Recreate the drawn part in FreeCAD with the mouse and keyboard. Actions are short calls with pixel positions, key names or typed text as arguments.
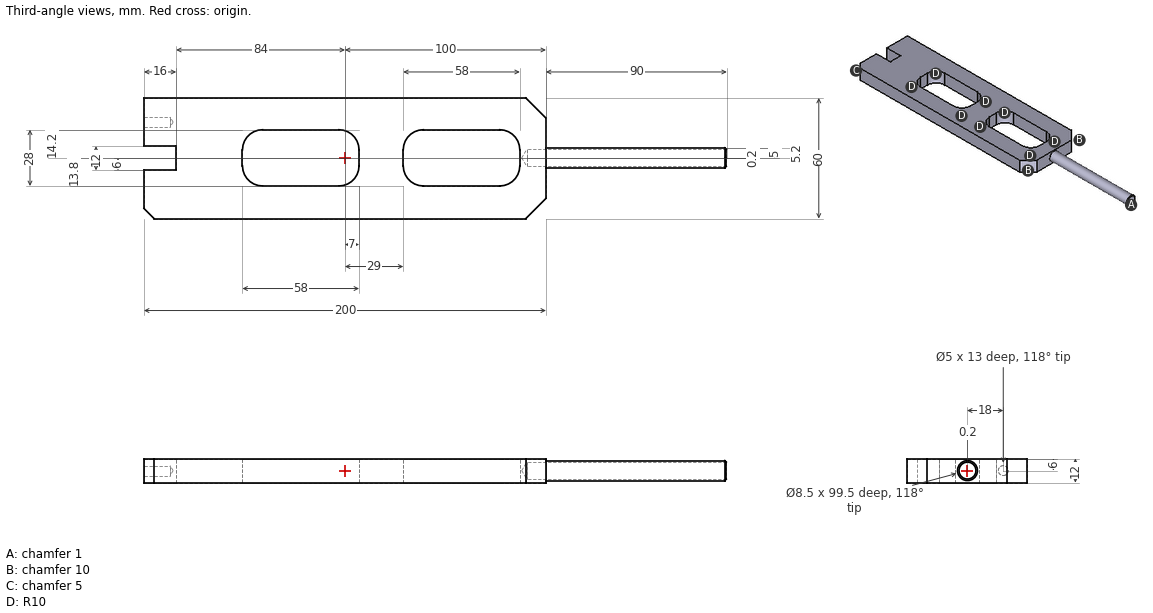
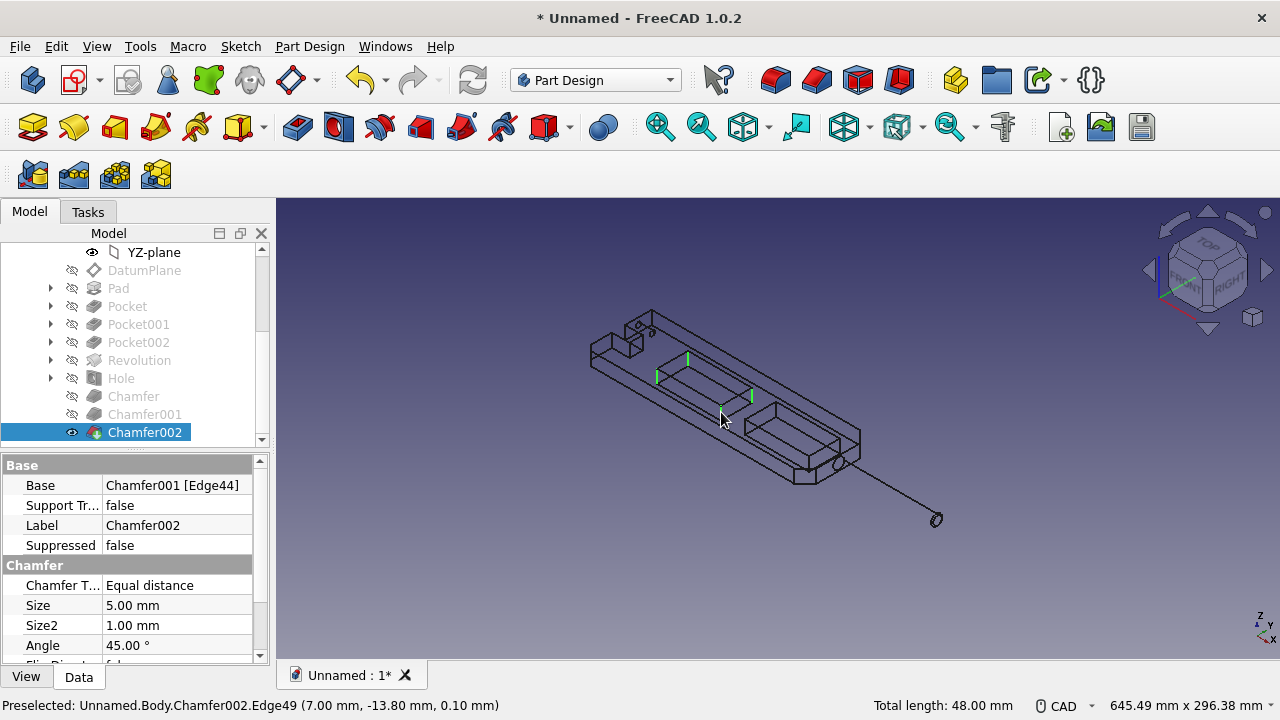
click(776, 410, ctrl)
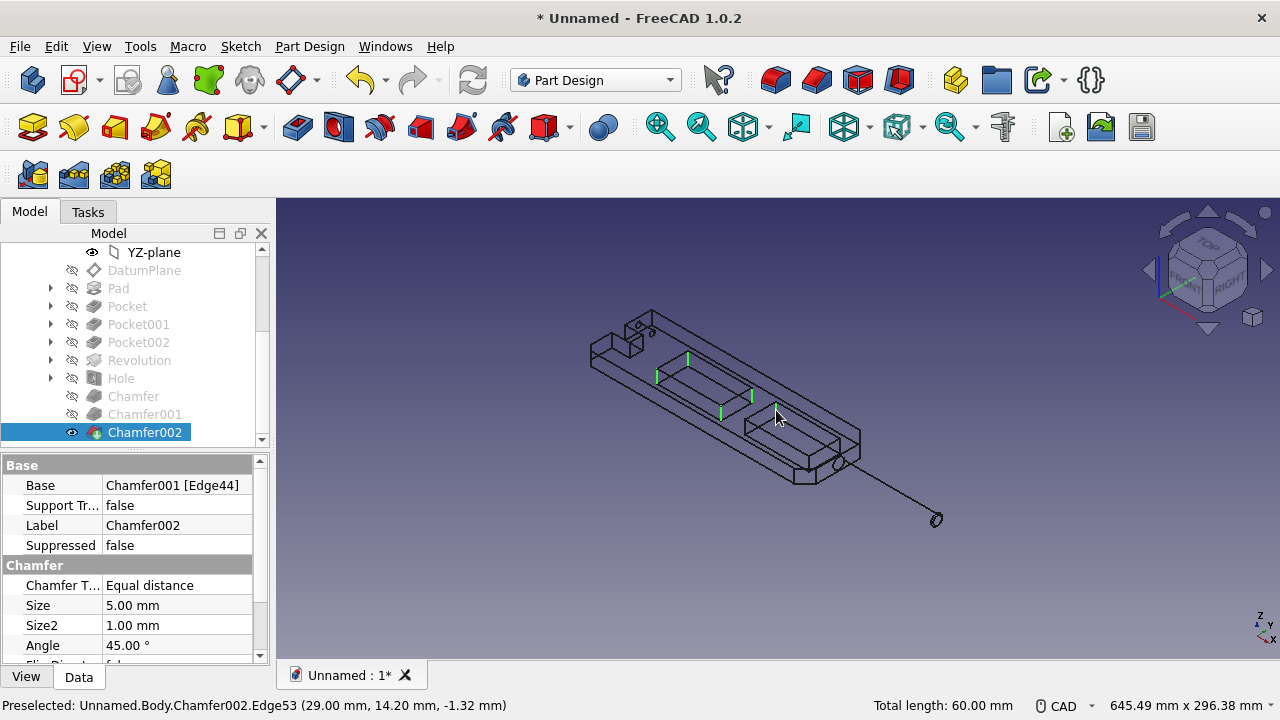
click(745, 426, ctrl)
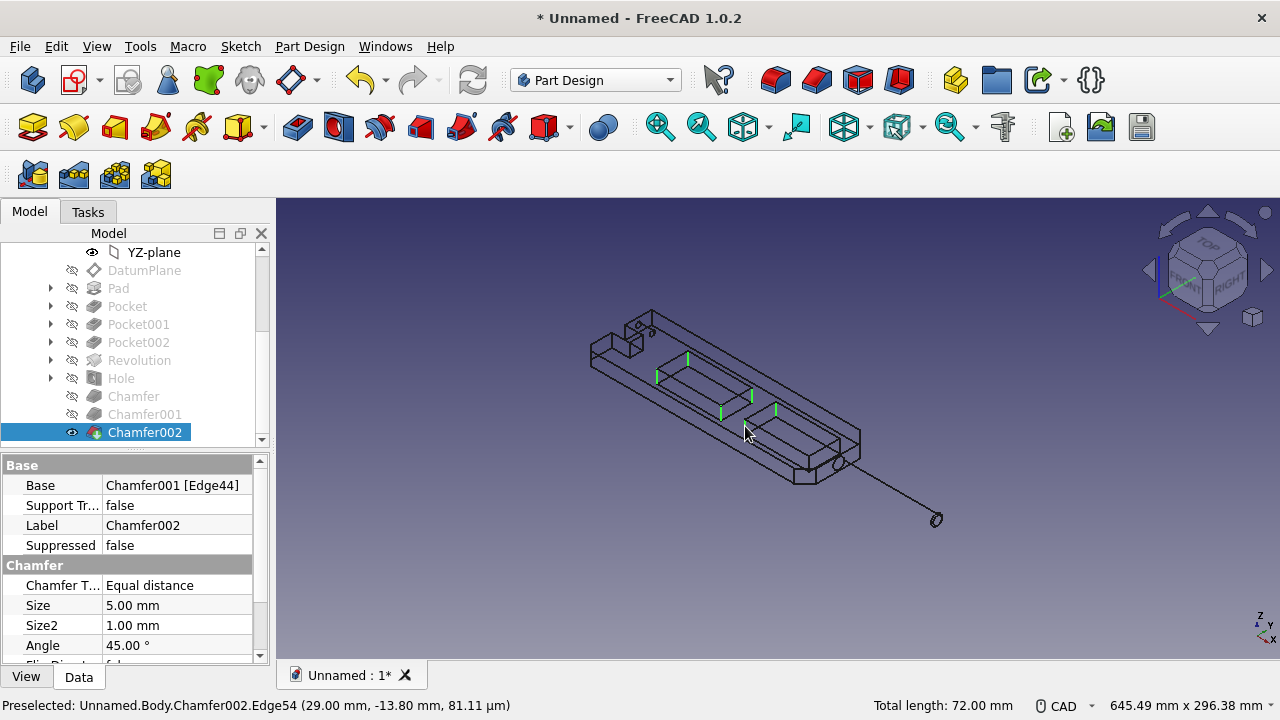
click(840, 445, ctrl)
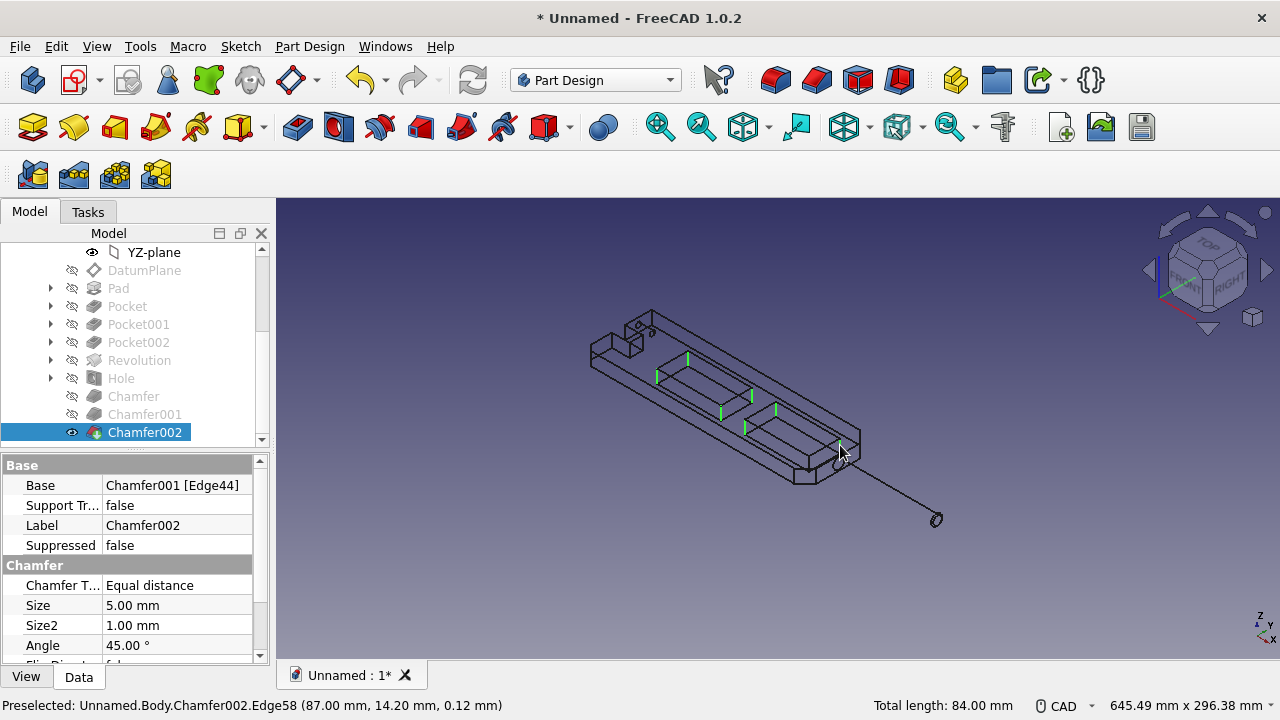
scroll(809, 463, up, 6)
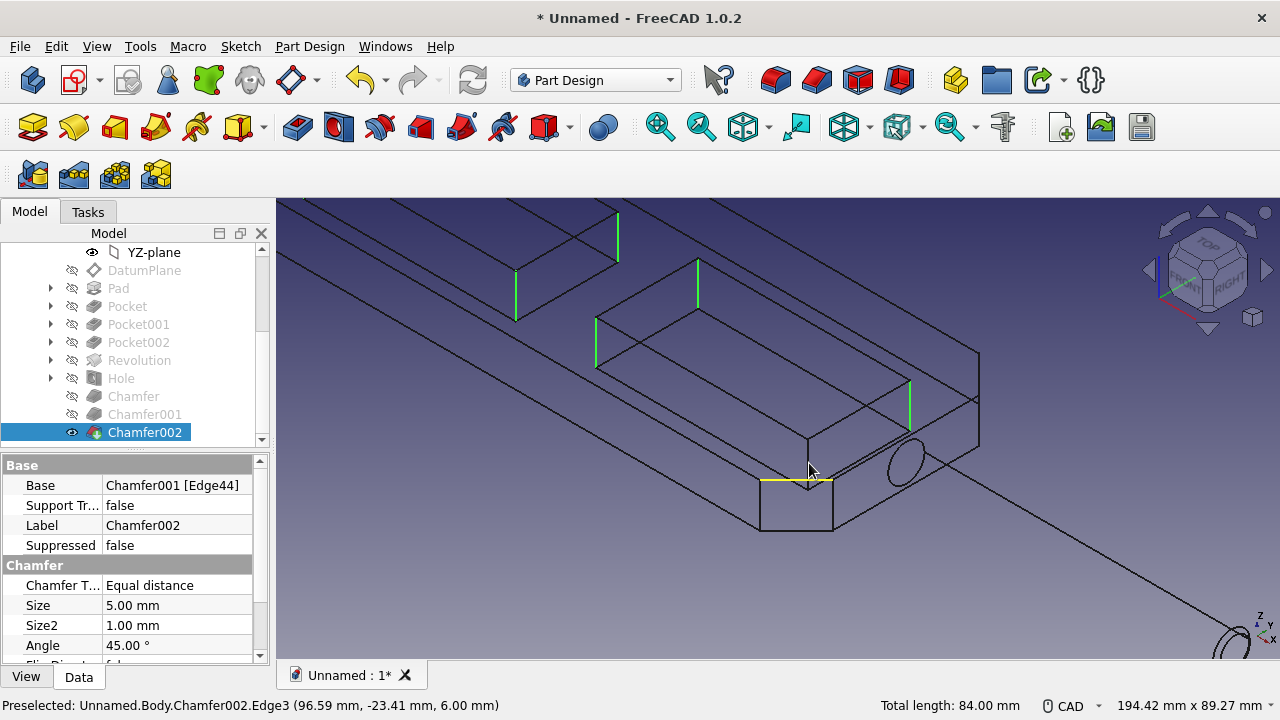
click(808, 464, ctrl)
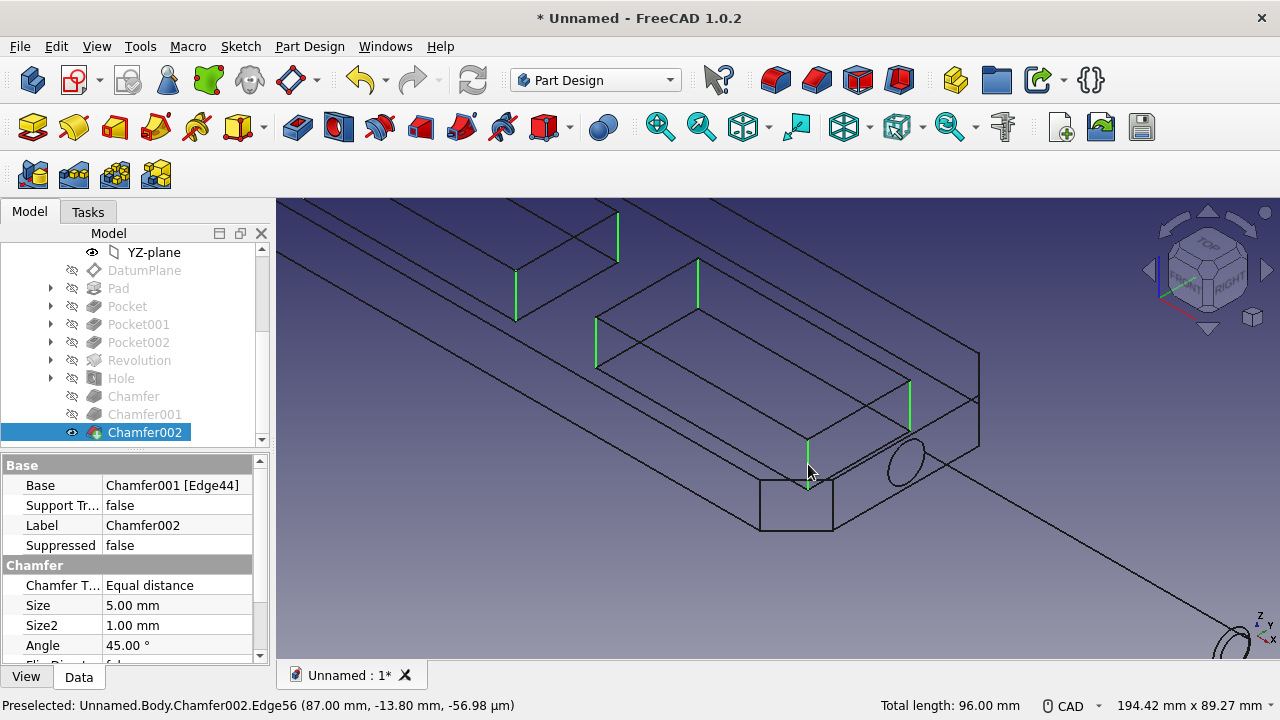
key(v)
key(1)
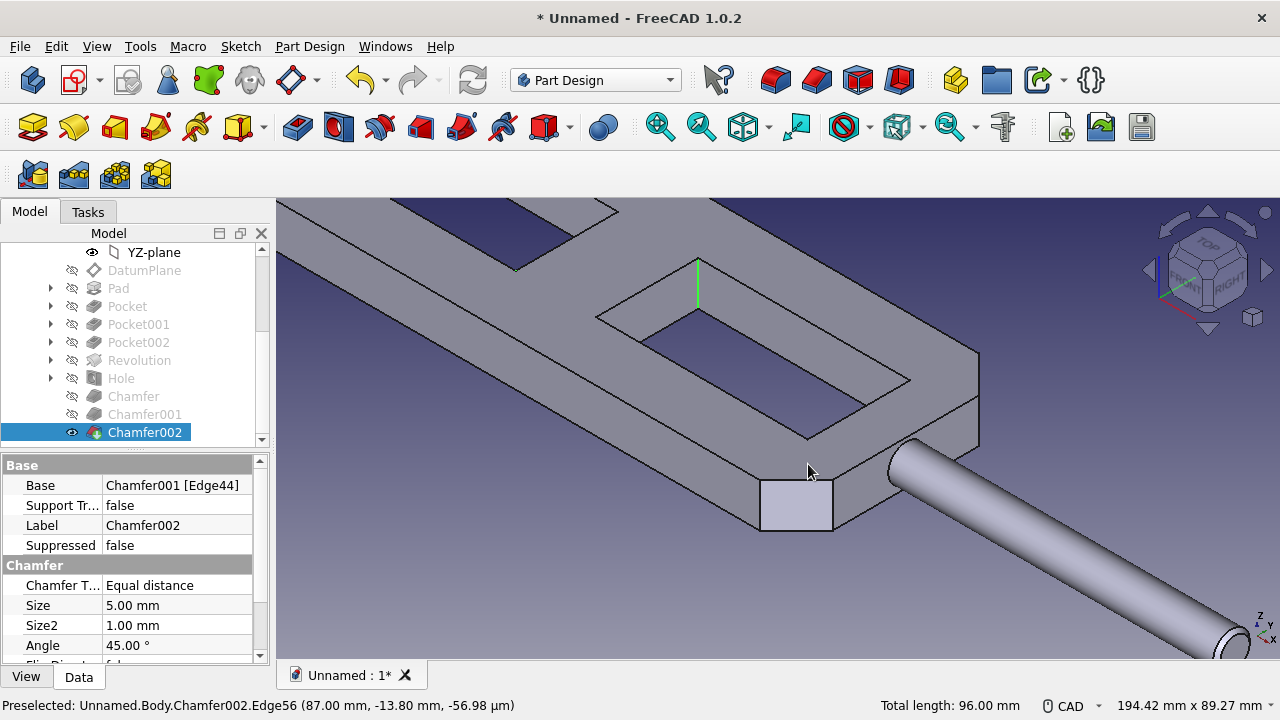
click(776, 80)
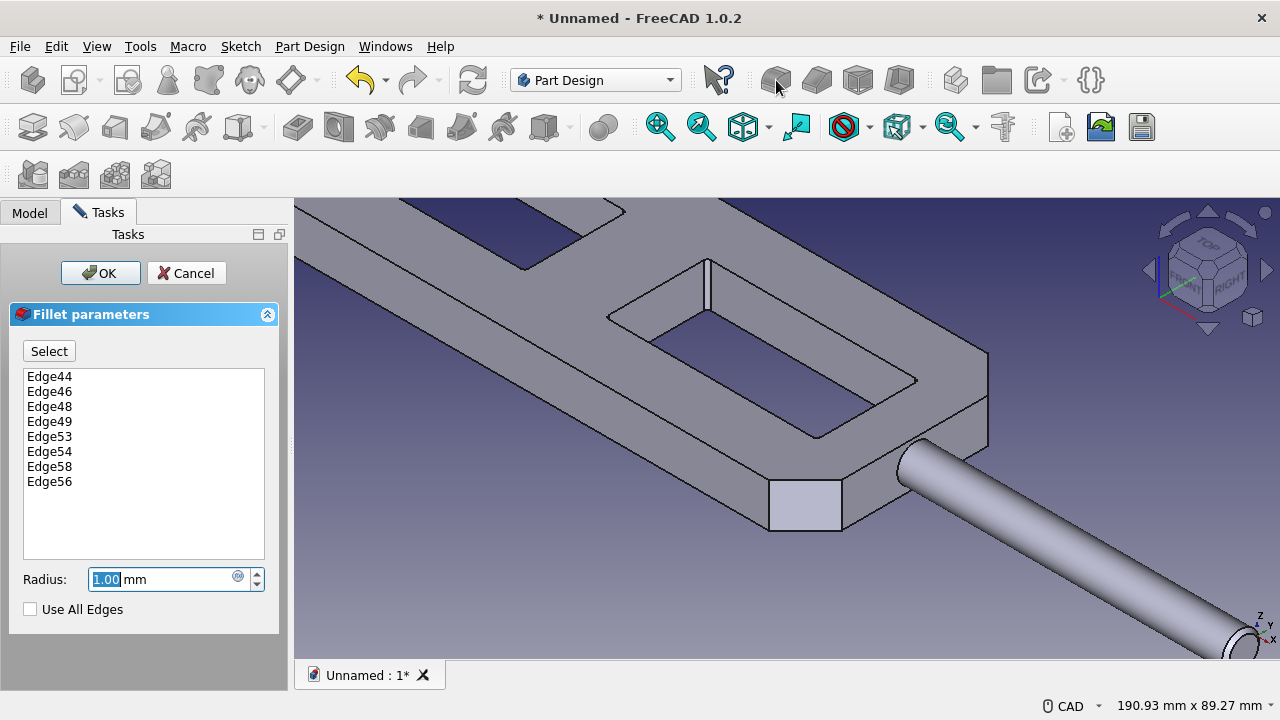
text(10)
key(Tab)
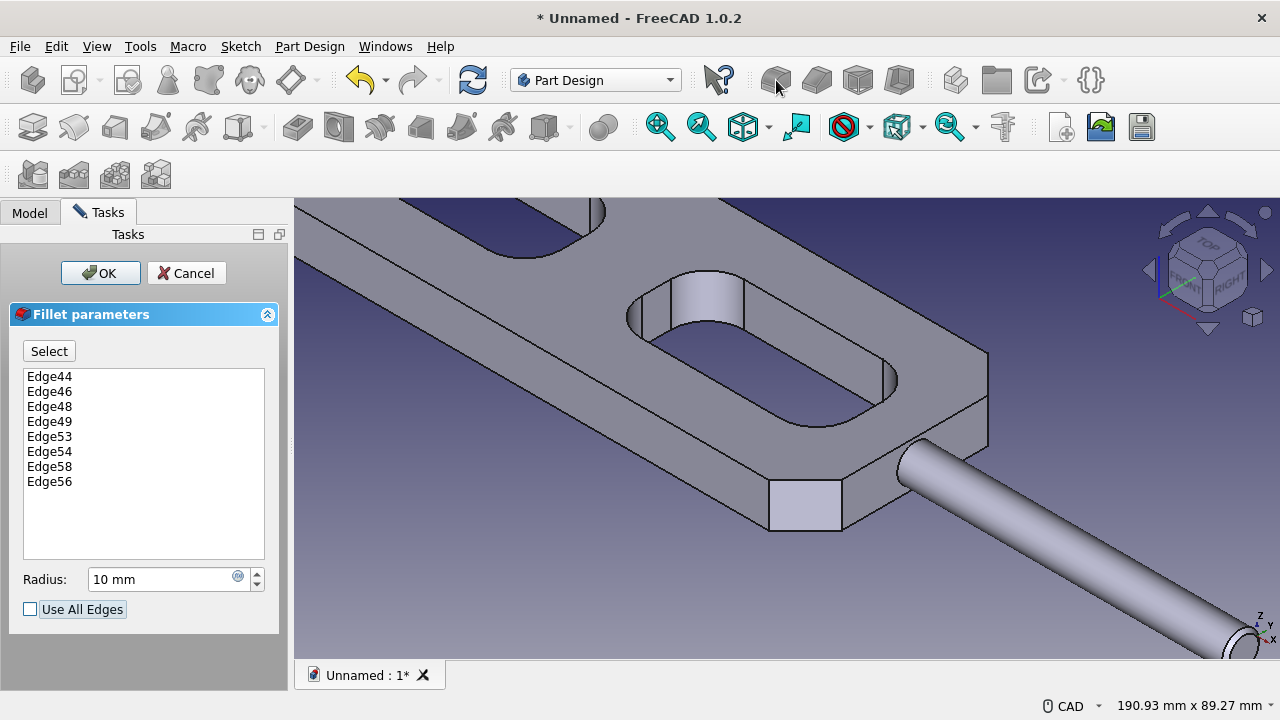
click(101, 273)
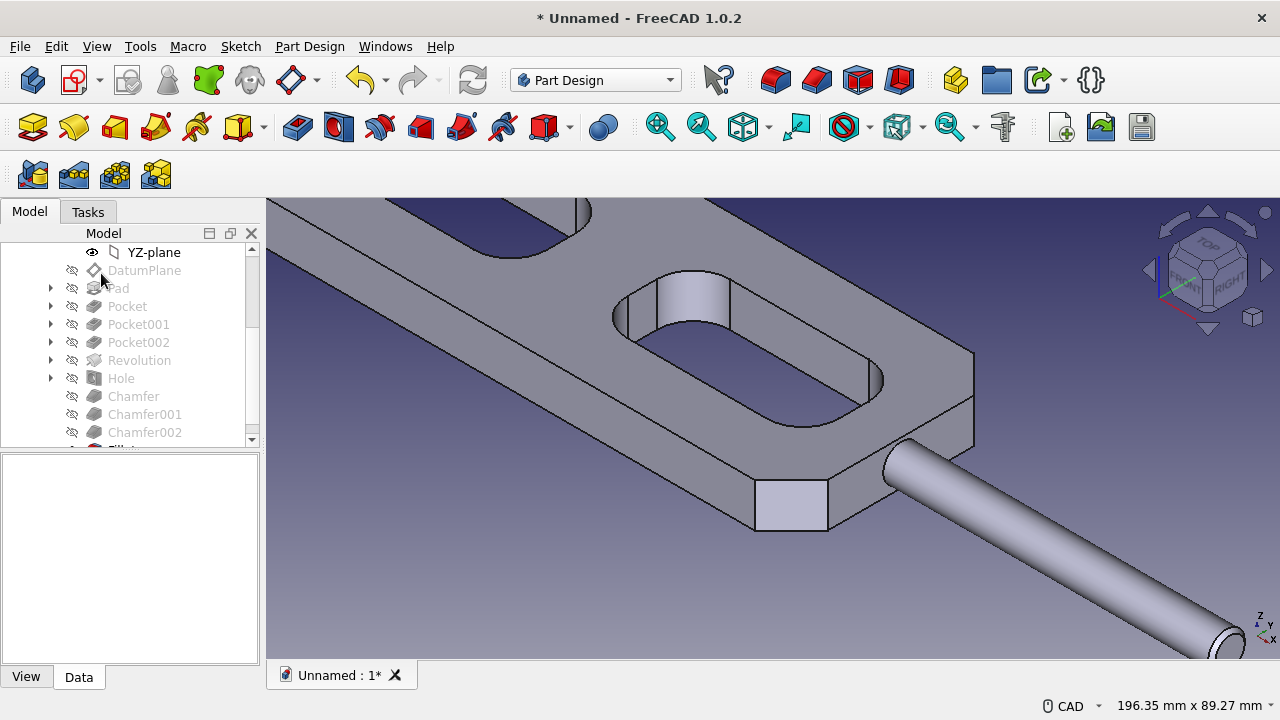
click(661, 128)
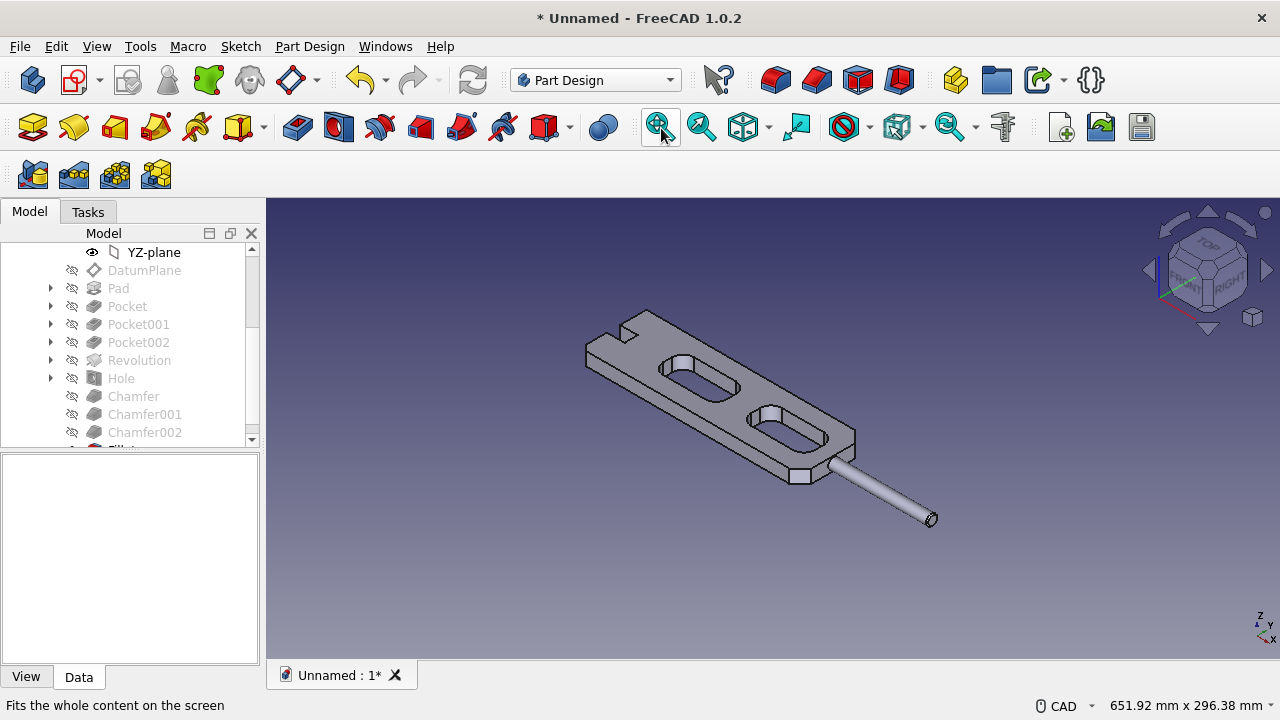
scroll(933, 519, up, 4)